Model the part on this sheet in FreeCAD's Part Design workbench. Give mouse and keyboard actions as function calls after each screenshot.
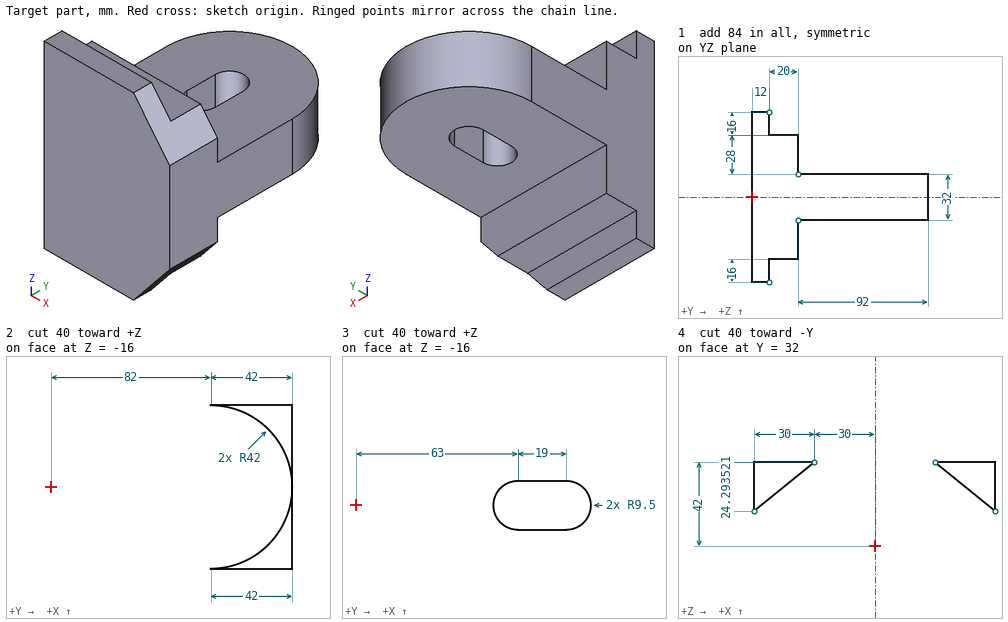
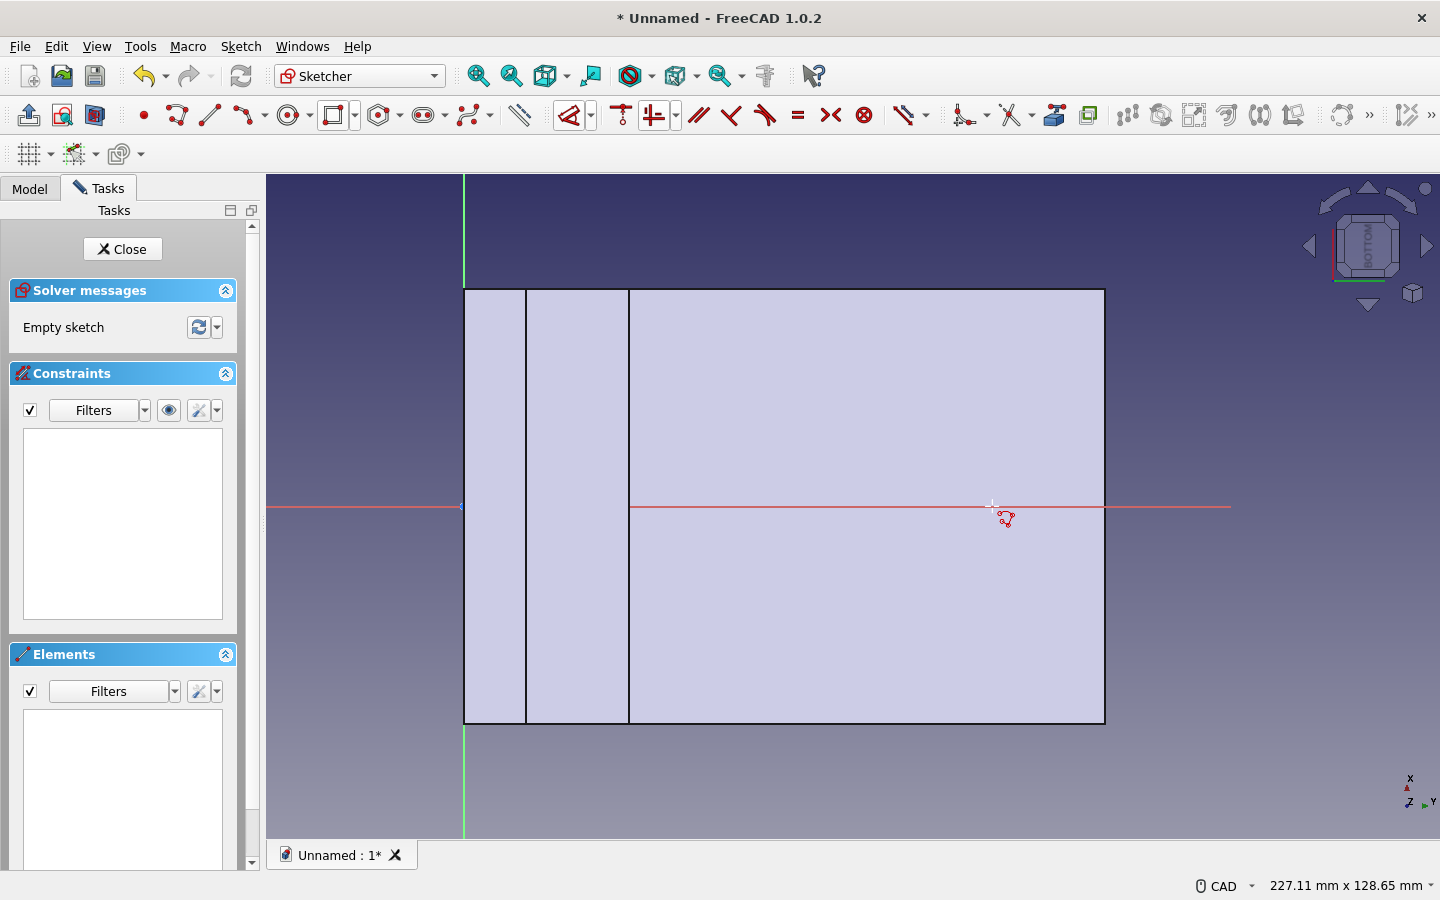
click(1105, 506)
click(1105, 289)
click(888, 289)
right_click(888, 289)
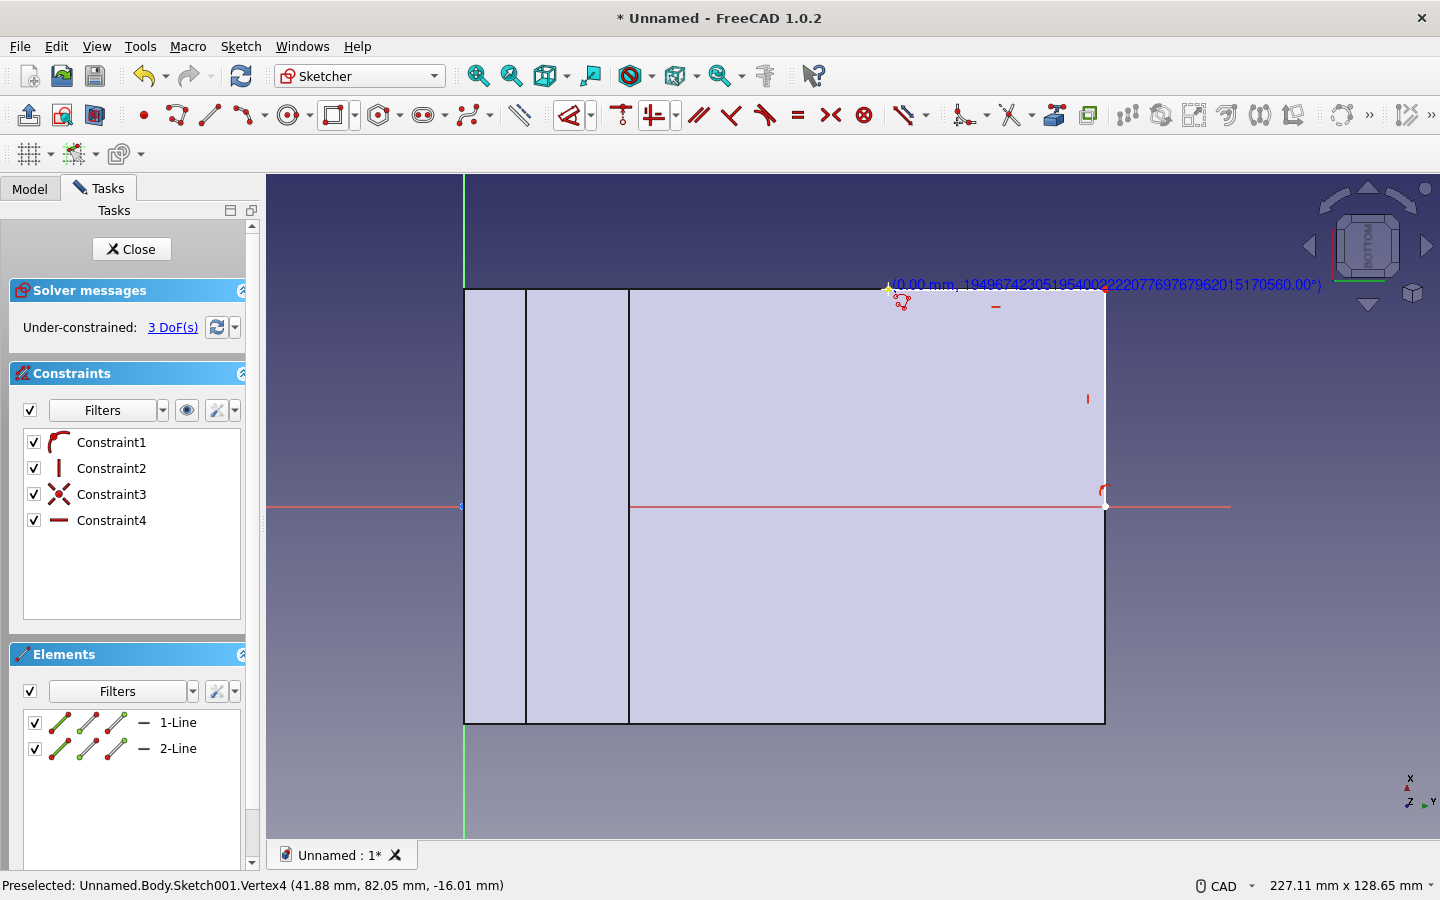
key(g)
key(3)
key(a)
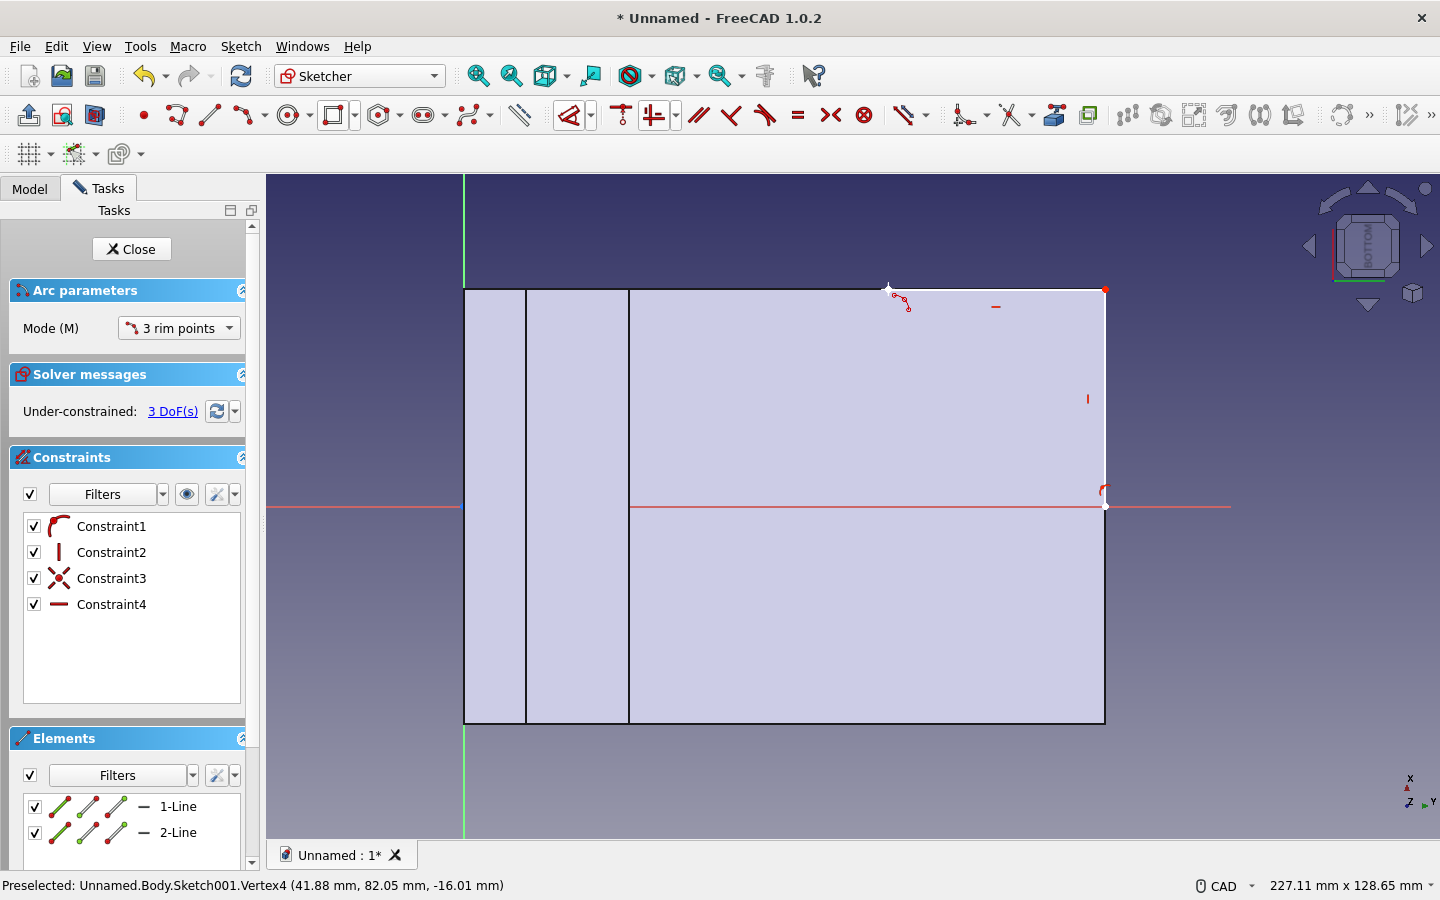
click(888, 290)
click(1105, 506)
click(1041, 353)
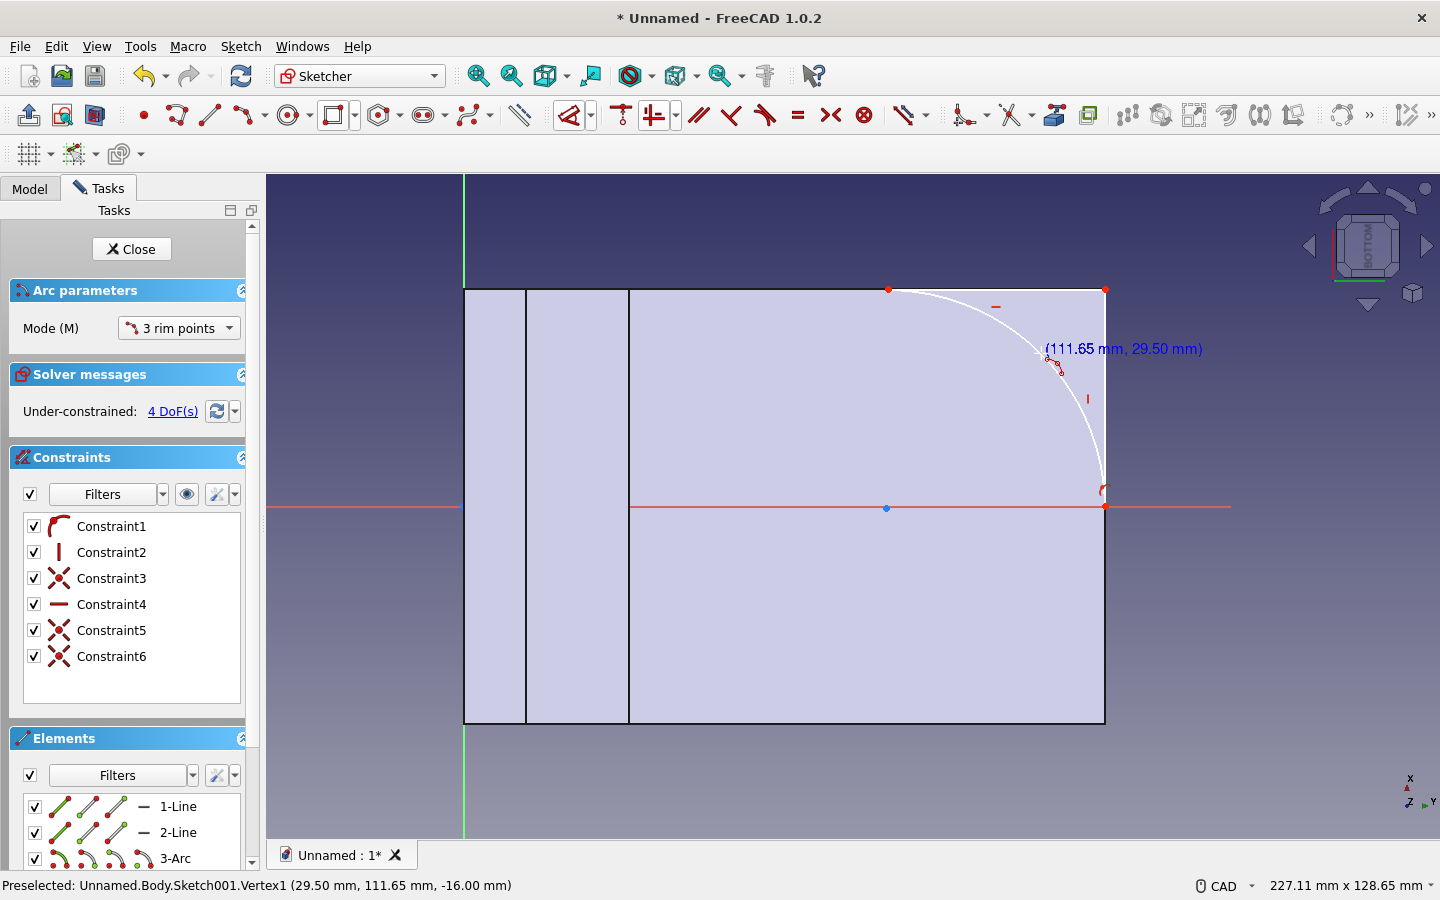
key(g)
key(m)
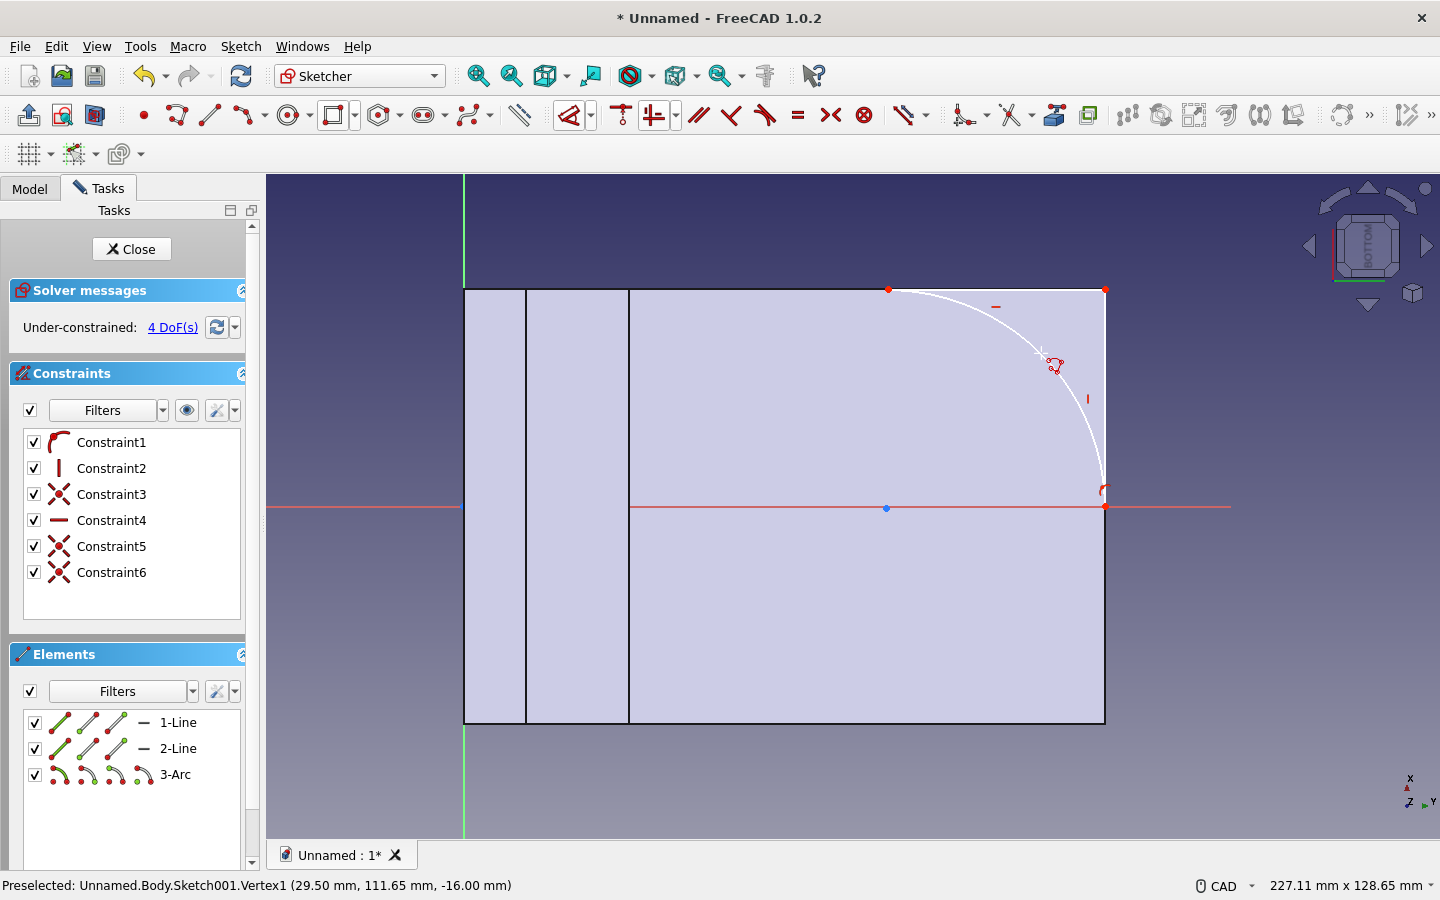
click(888, 724)
click(1105, 724)
click(1105, 506)
right_click(1105, 724)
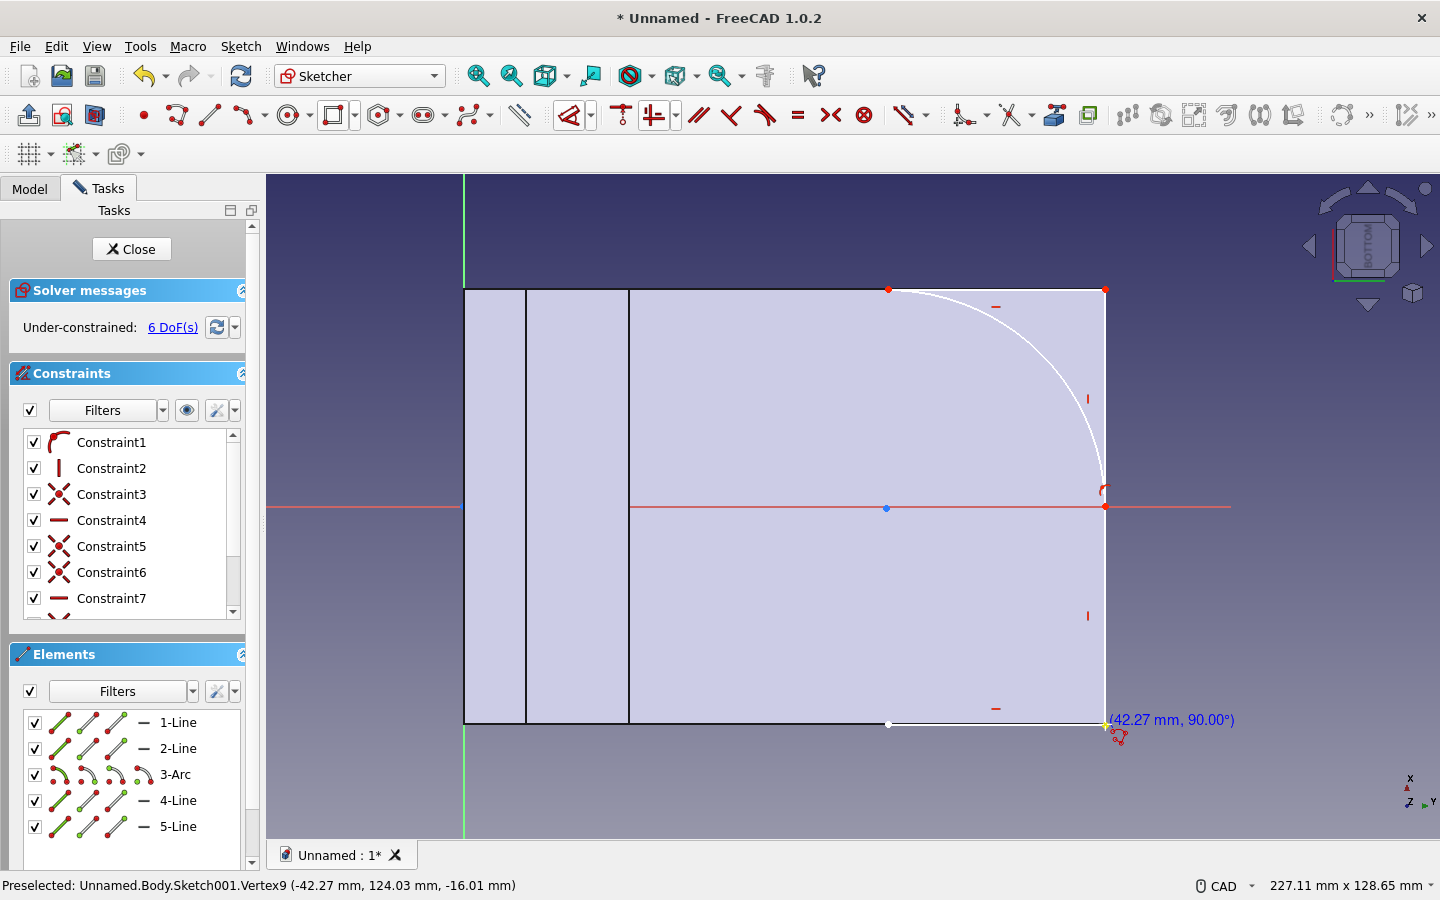
click(242, 116)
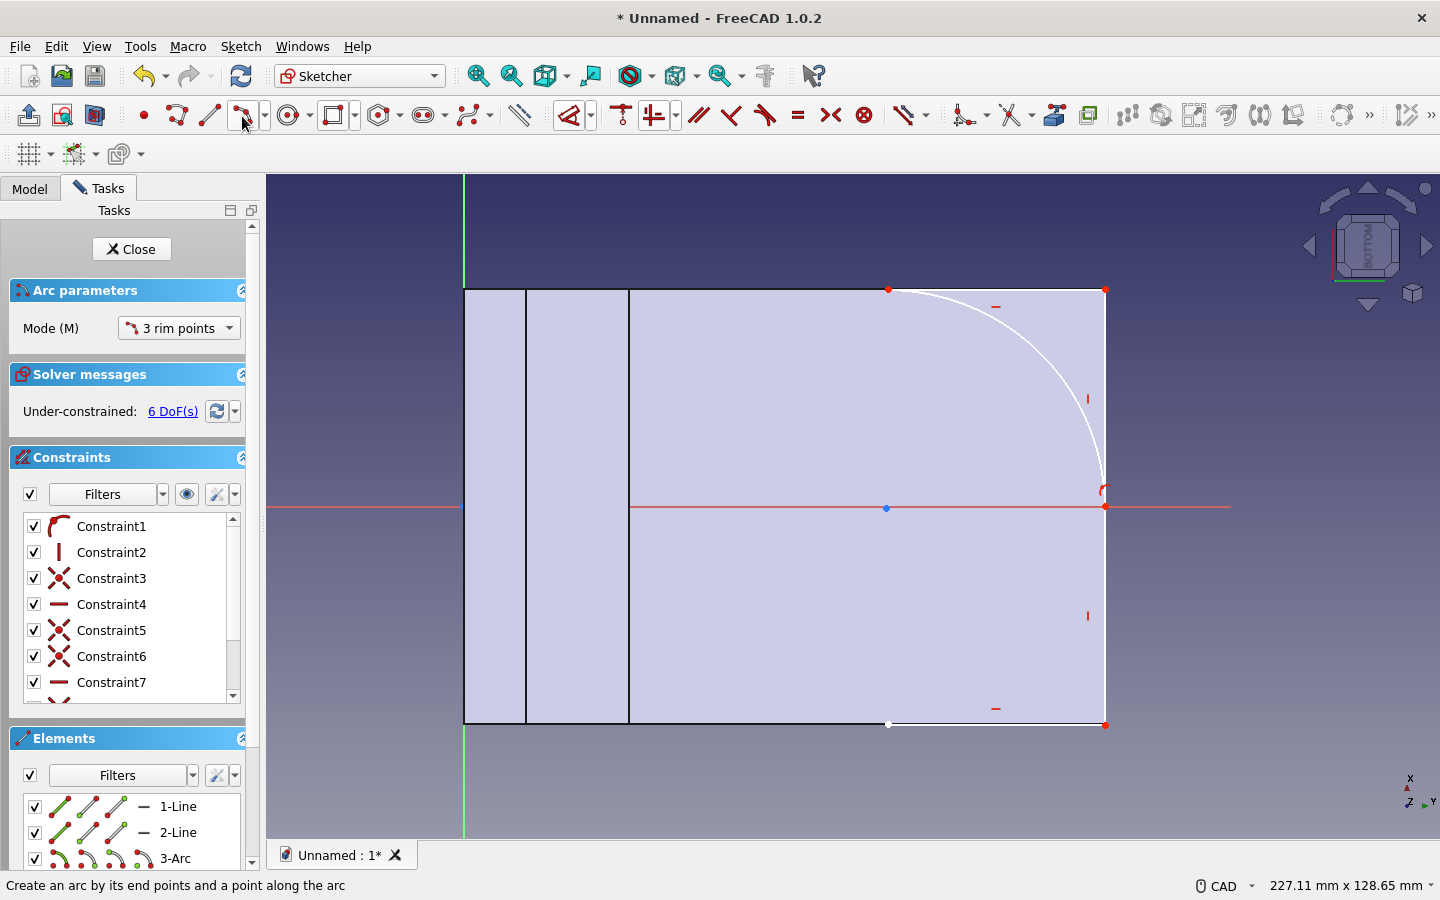
click(1105, 506)
click(888, 725)
click(1041, 660)
key(Escape)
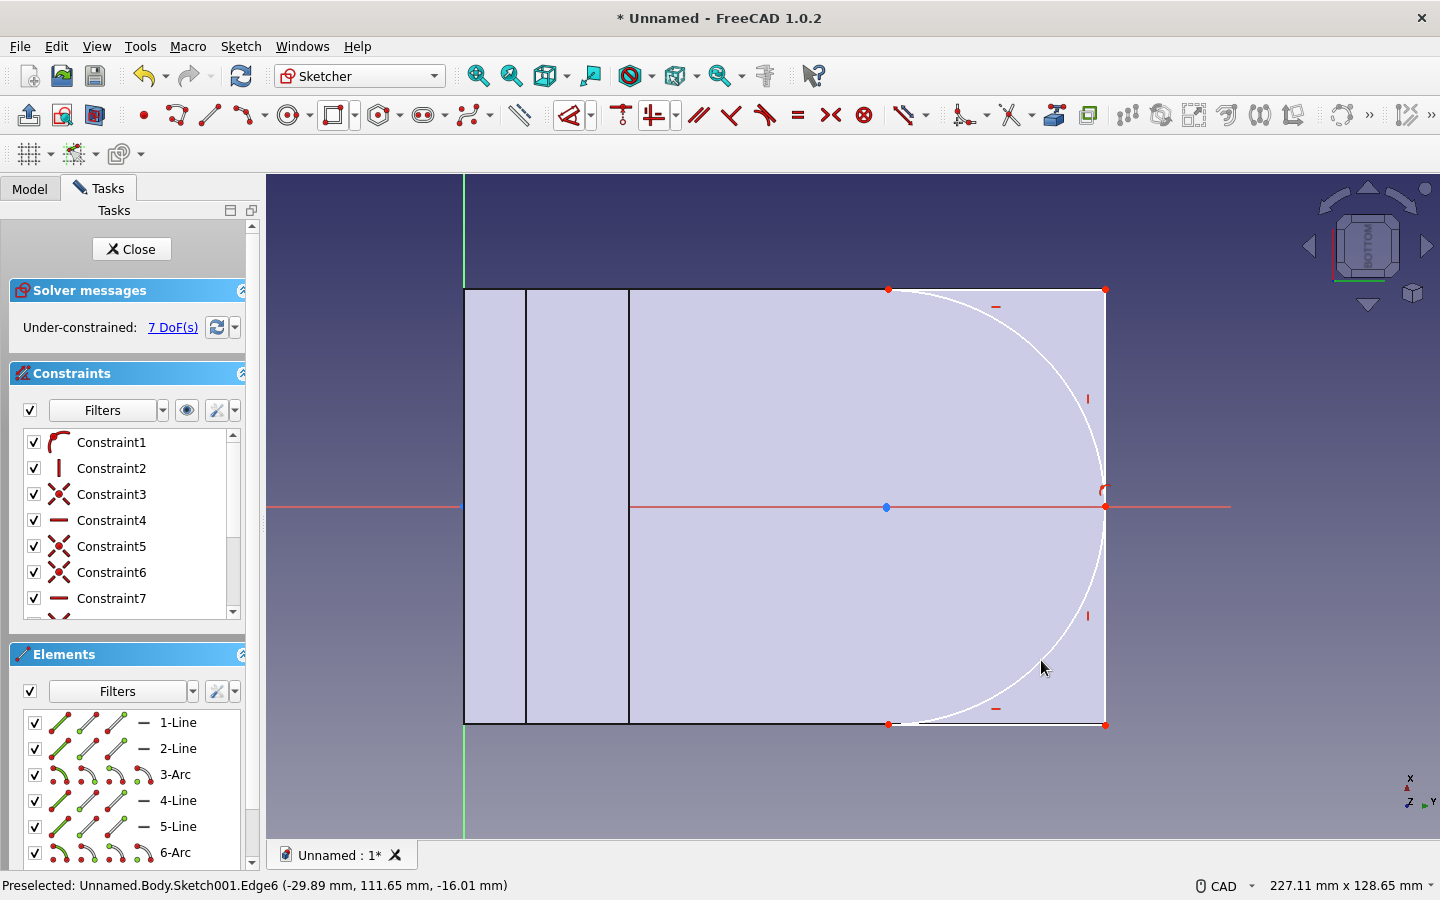
click(1081, 408)